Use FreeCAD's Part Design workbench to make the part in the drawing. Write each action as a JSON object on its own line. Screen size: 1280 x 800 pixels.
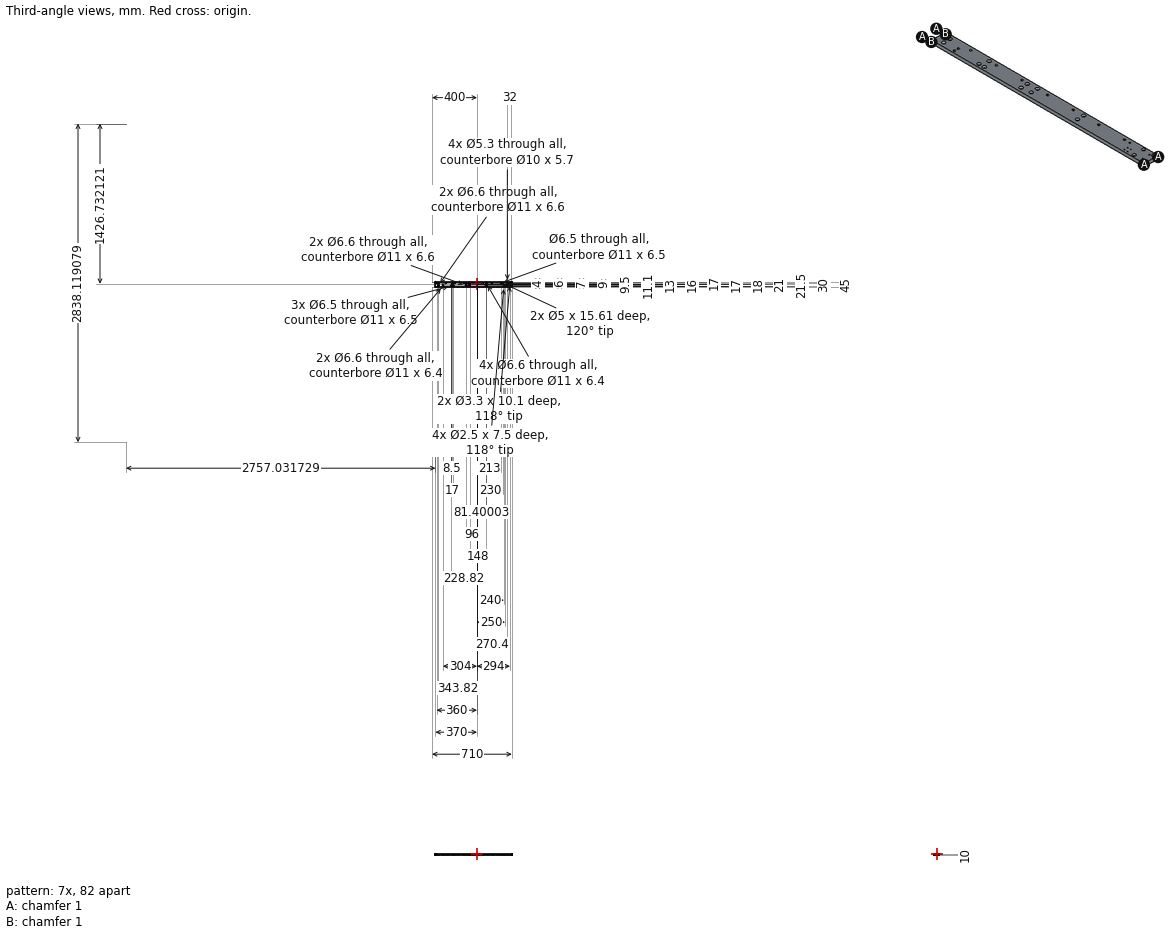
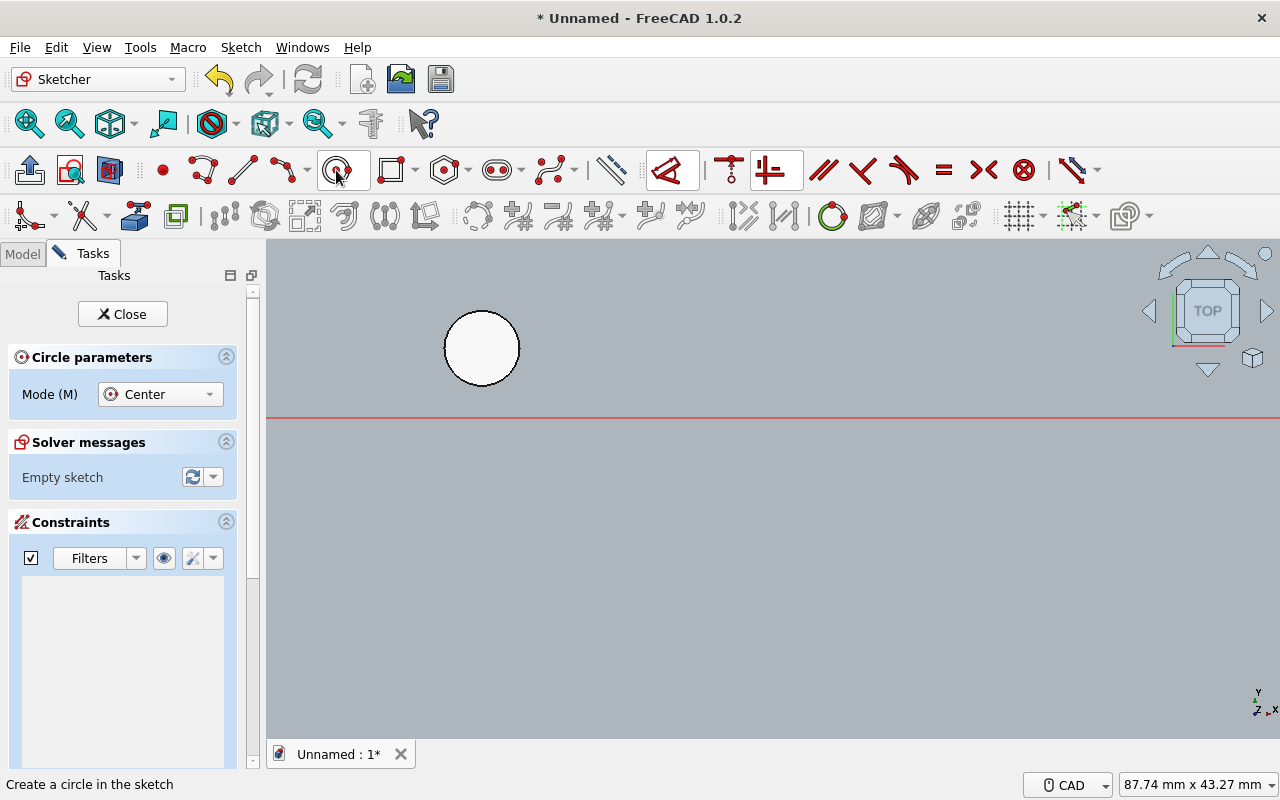
{"action": "left_click", "coordinate": [702, 603]}
{"action": "left_click", "coordinate": [728, 576]}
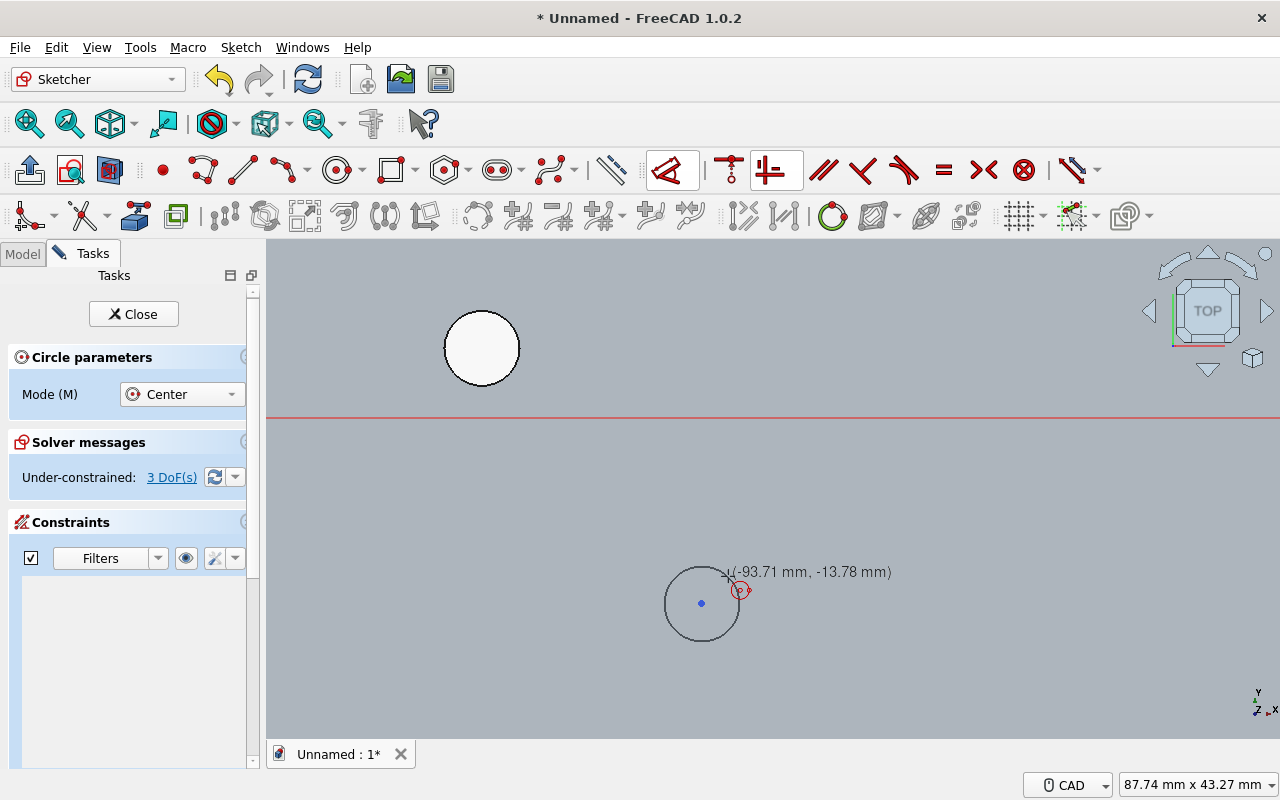
{"action": "left_click", "coordinate": [702, 371]}
{"action": "left_click", "coordinate": [728, 345]}
{"action": "key", "text": "Escape"}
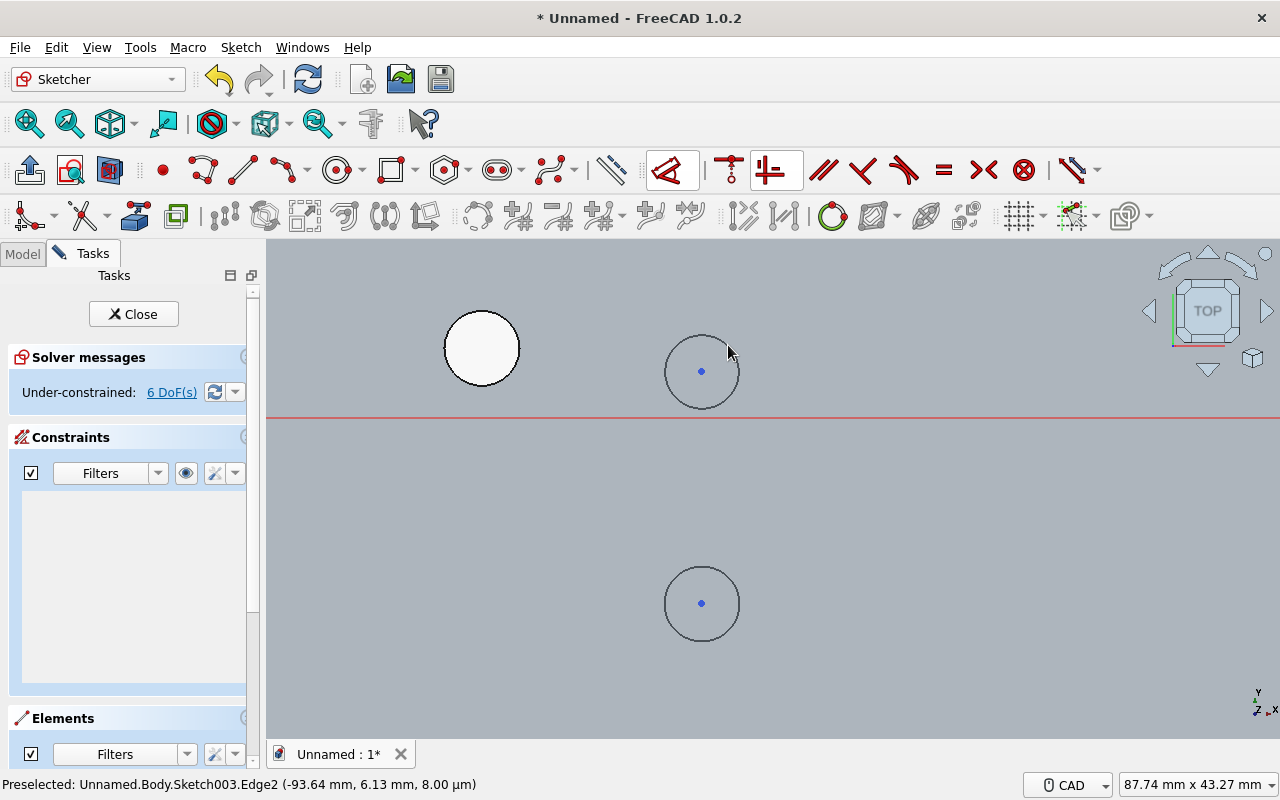
{"action": "left_click", "coordinate": [728, 577]}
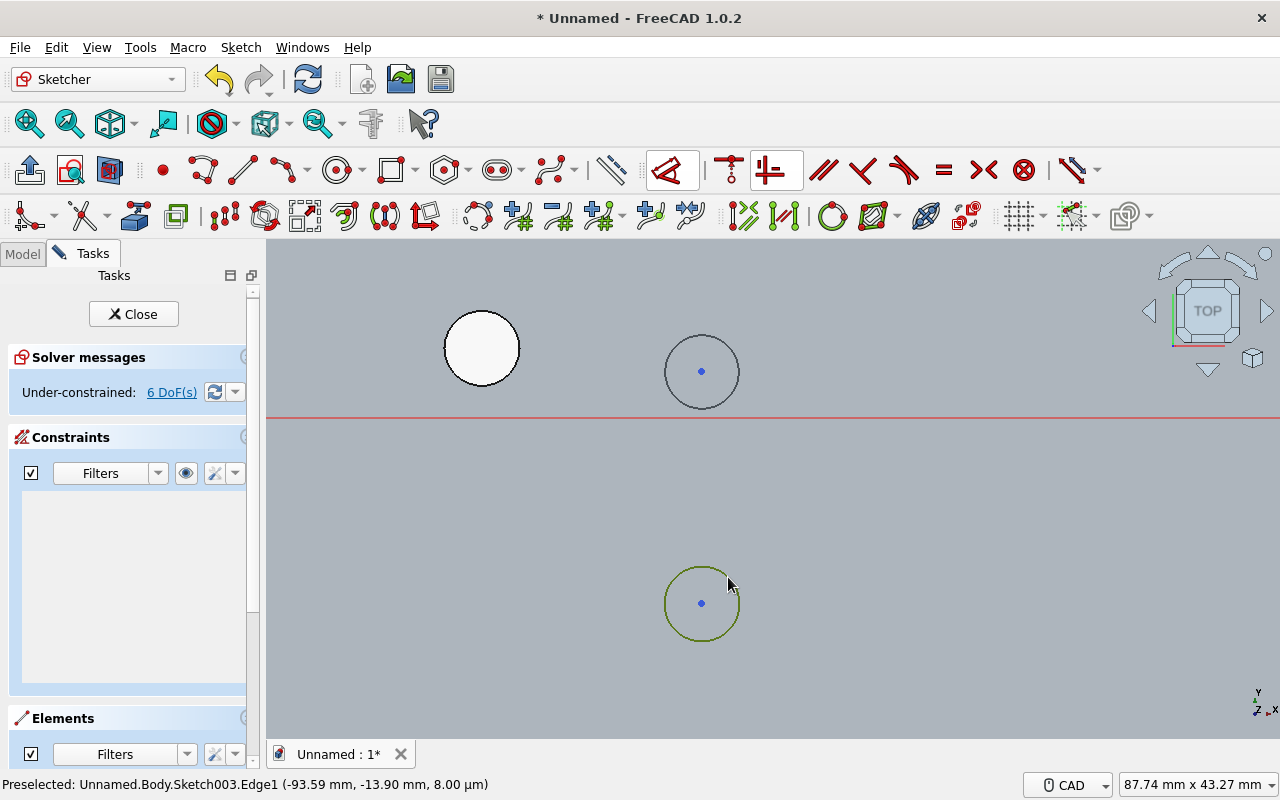
{"action": "left_click", "coordinate": [728, 346]}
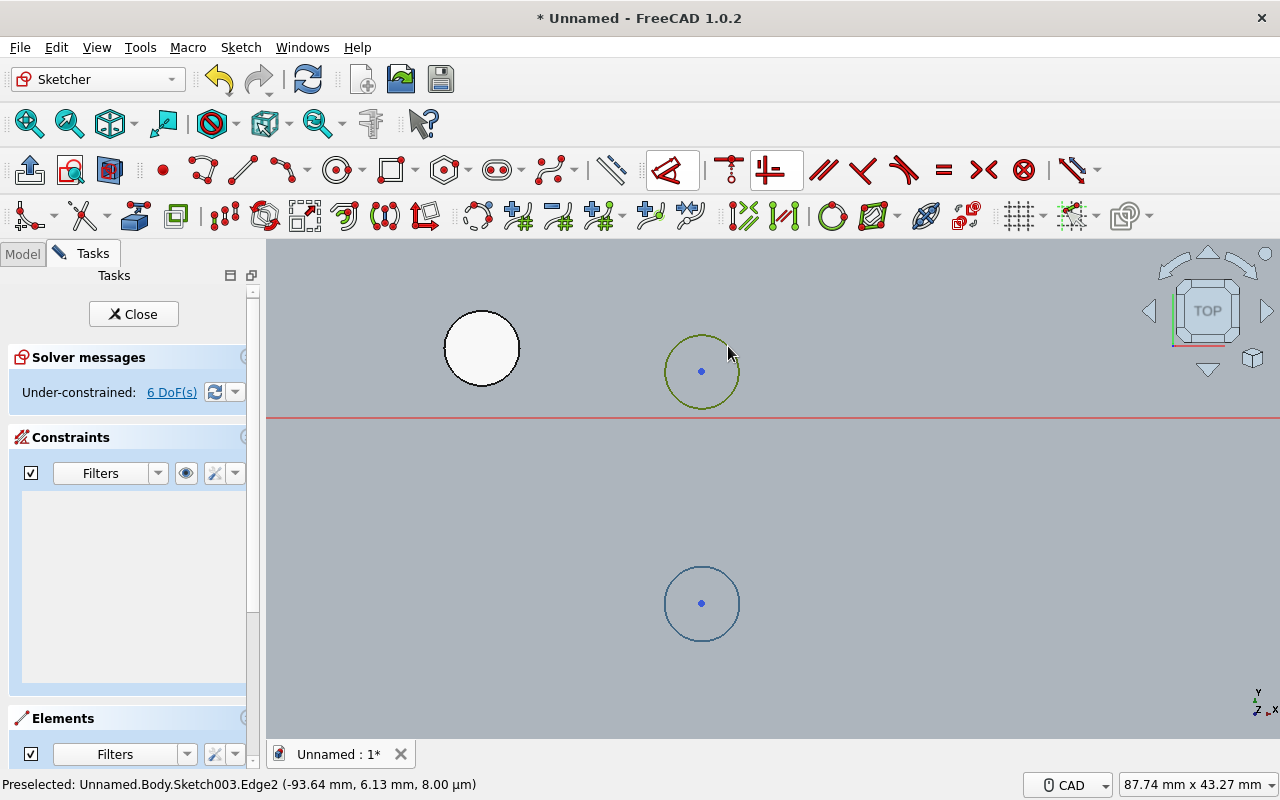
{"action": "left_click", "coordinate": [944, 170]}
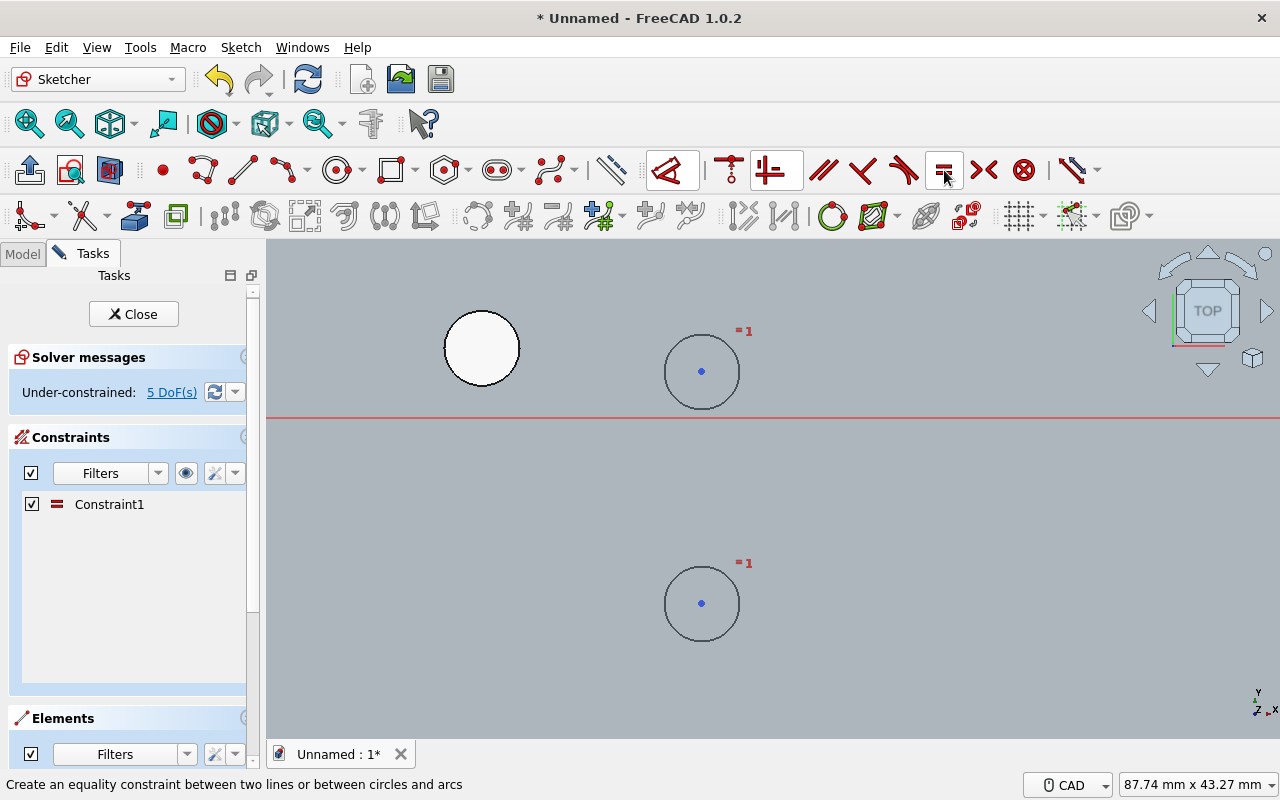
{"action": "left_click", "coordinate": [702, 604]}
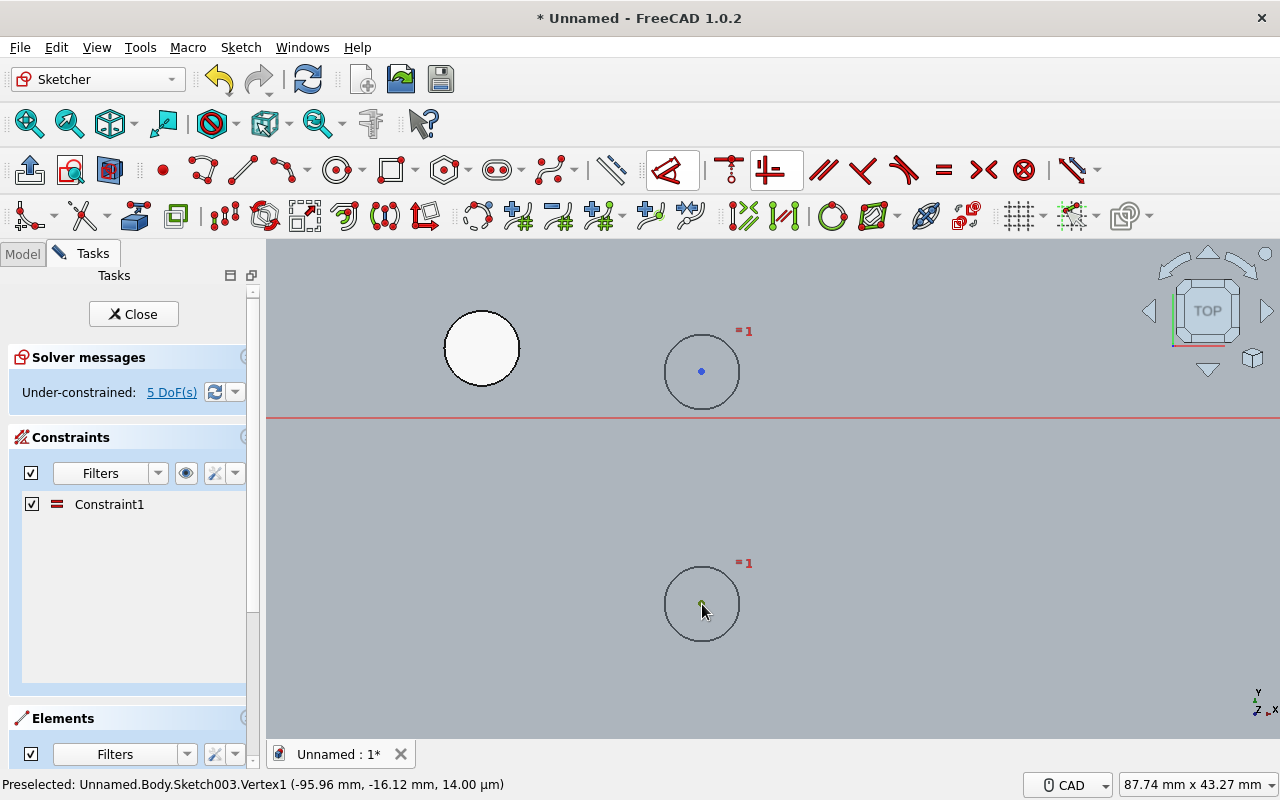
{"action": "left_click", "coordinate": [702, 372]}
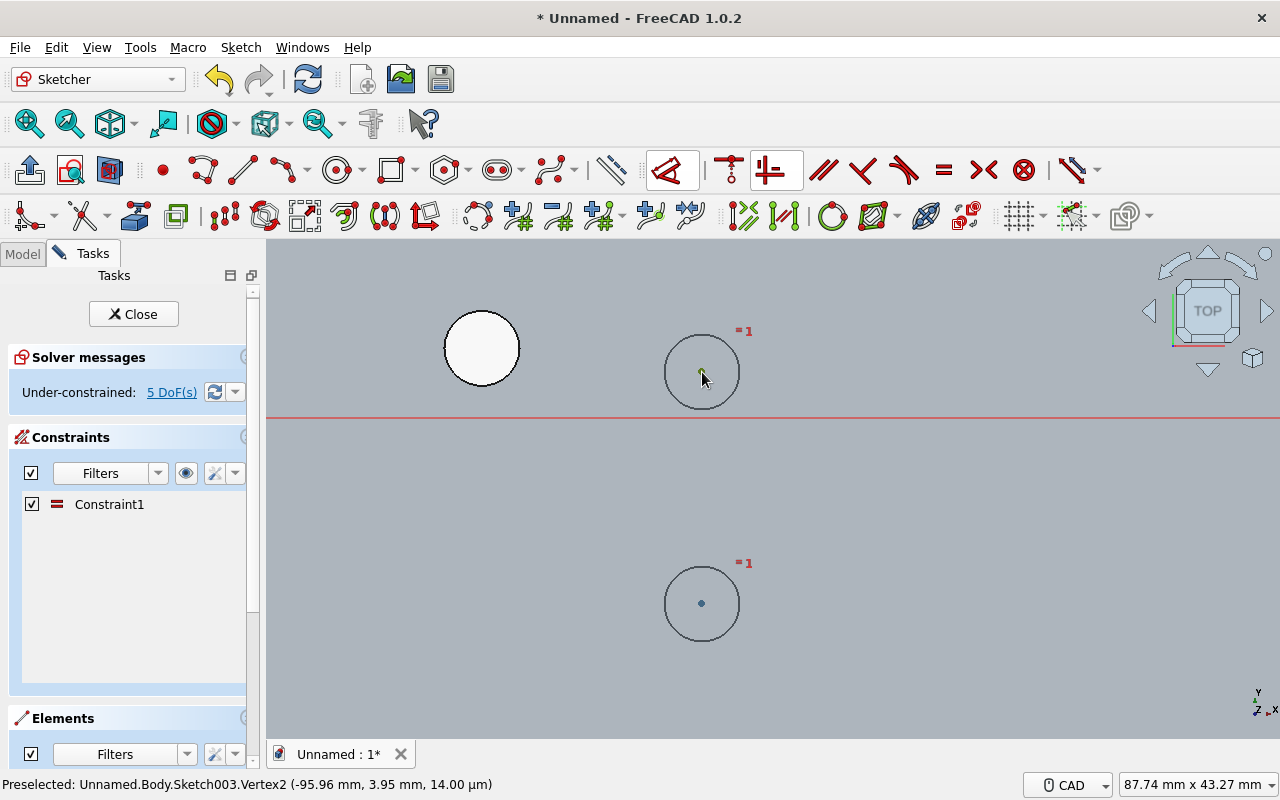
{"action": "left_click", "coordinate": [798, 170]}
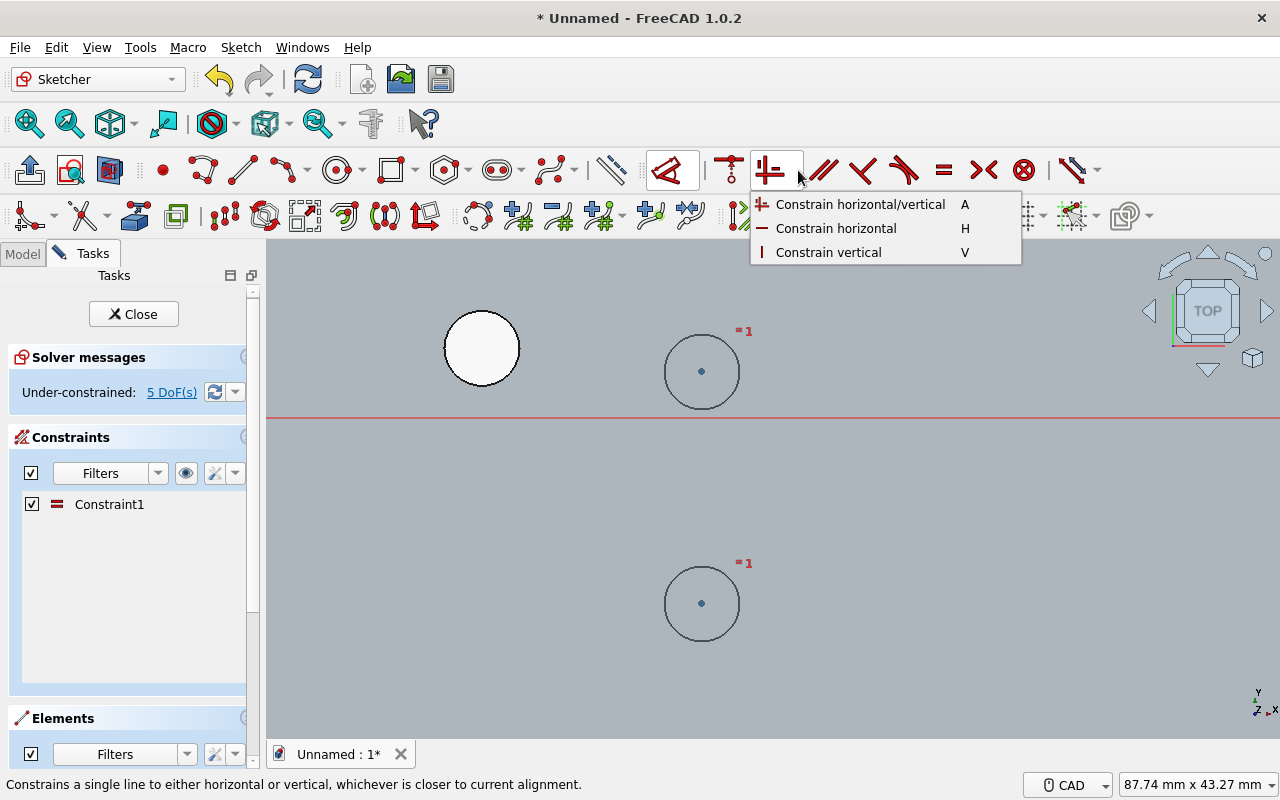
{"action": "left_click", "coordinate": [886, 252]}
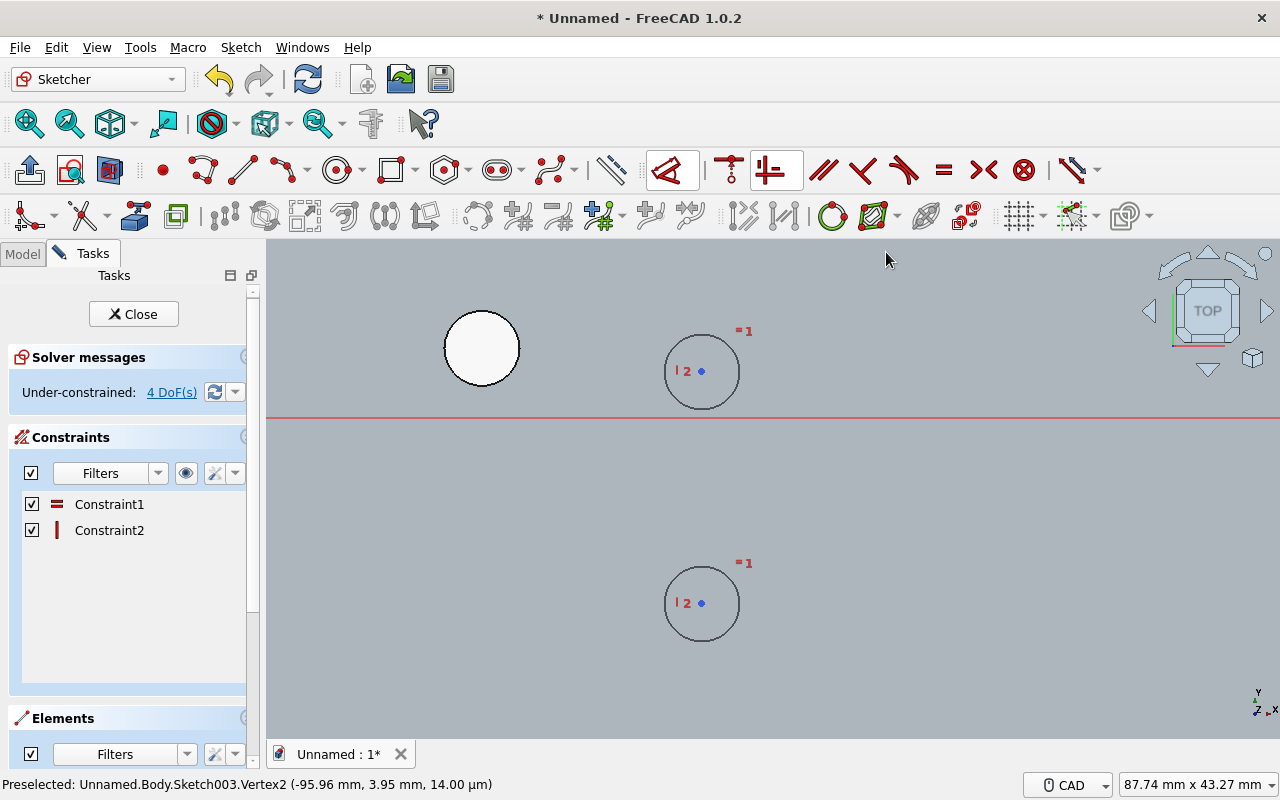
{"action": "left_click", "coordinate": [728, 577]}